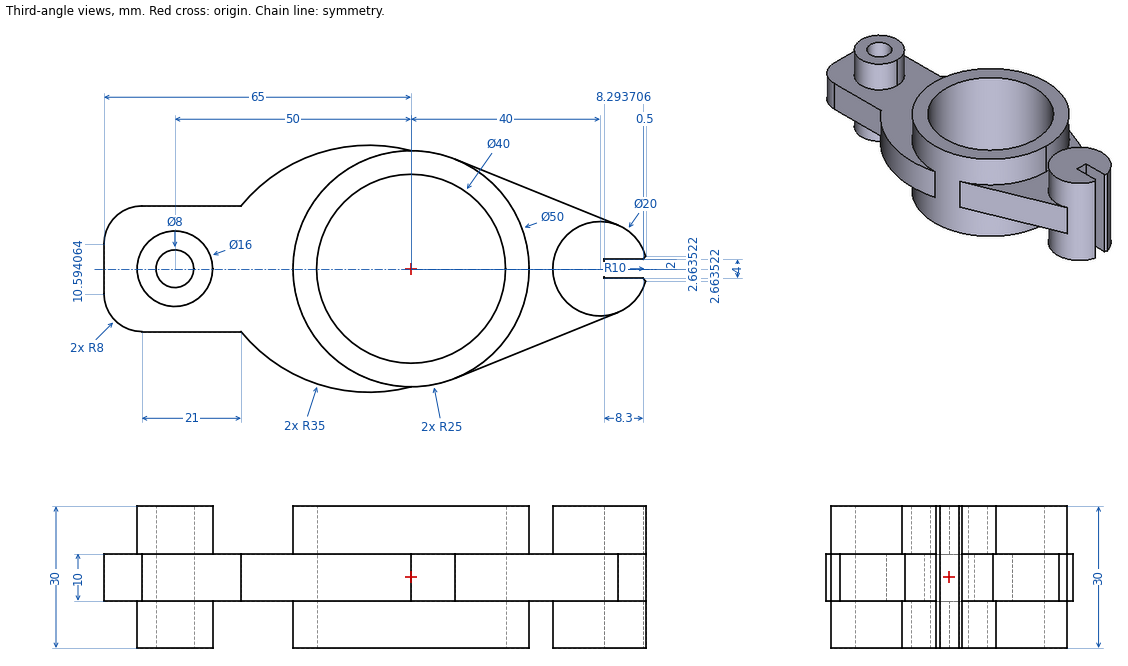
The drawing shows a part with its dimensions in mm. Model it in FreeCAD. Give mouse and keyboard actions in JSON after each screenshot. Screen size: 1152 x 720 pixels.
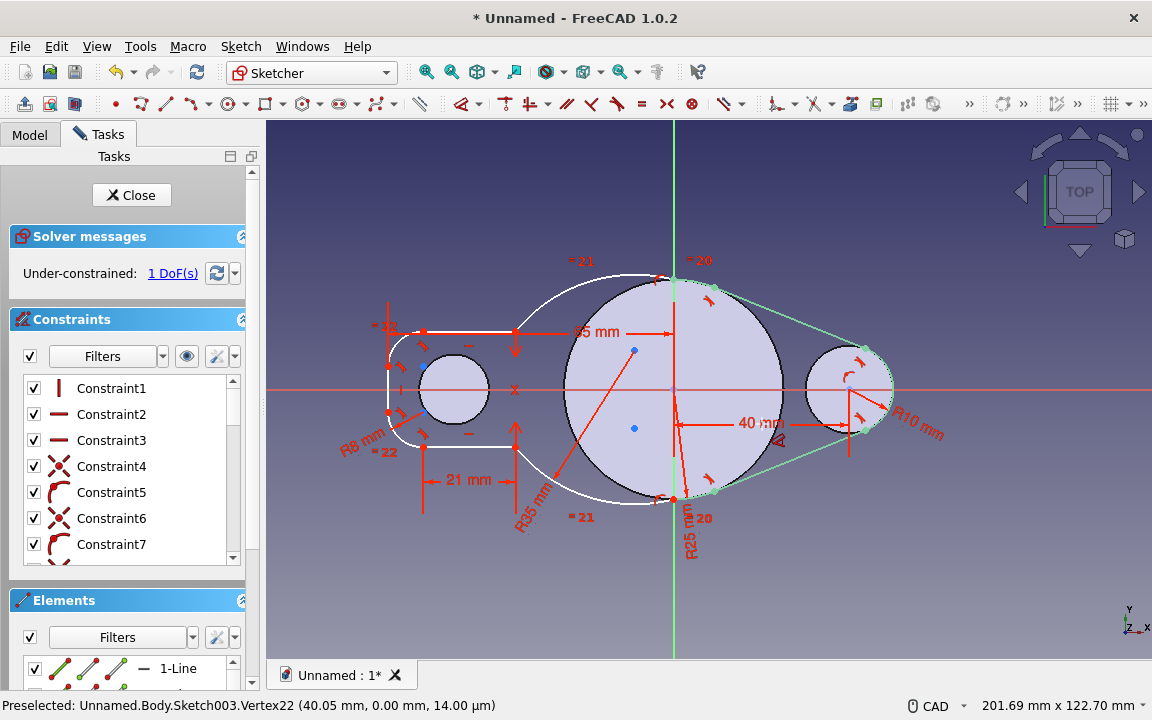
{"action": "scroll", "coordinate": [388, 380], "scroll_direction": "up", "scroll_amount": 3}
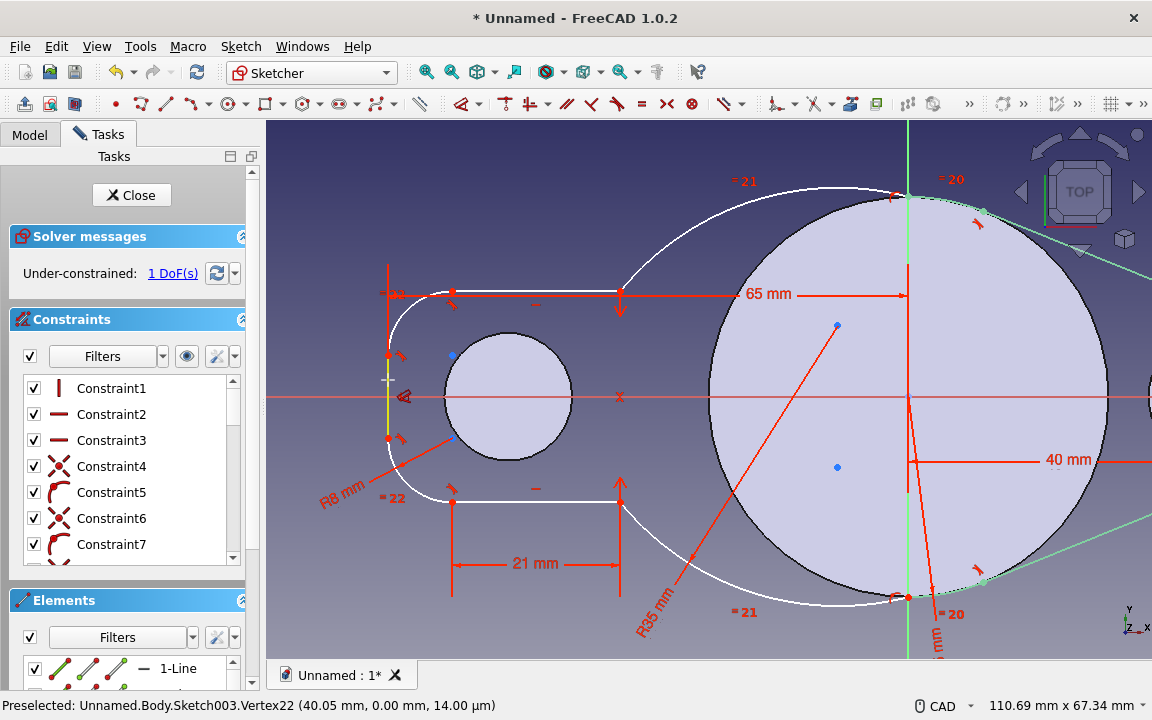
{"action": "left_click", "coordinate": [388, 380]}
{"action": "left_click", "coordinate": [354, 378]}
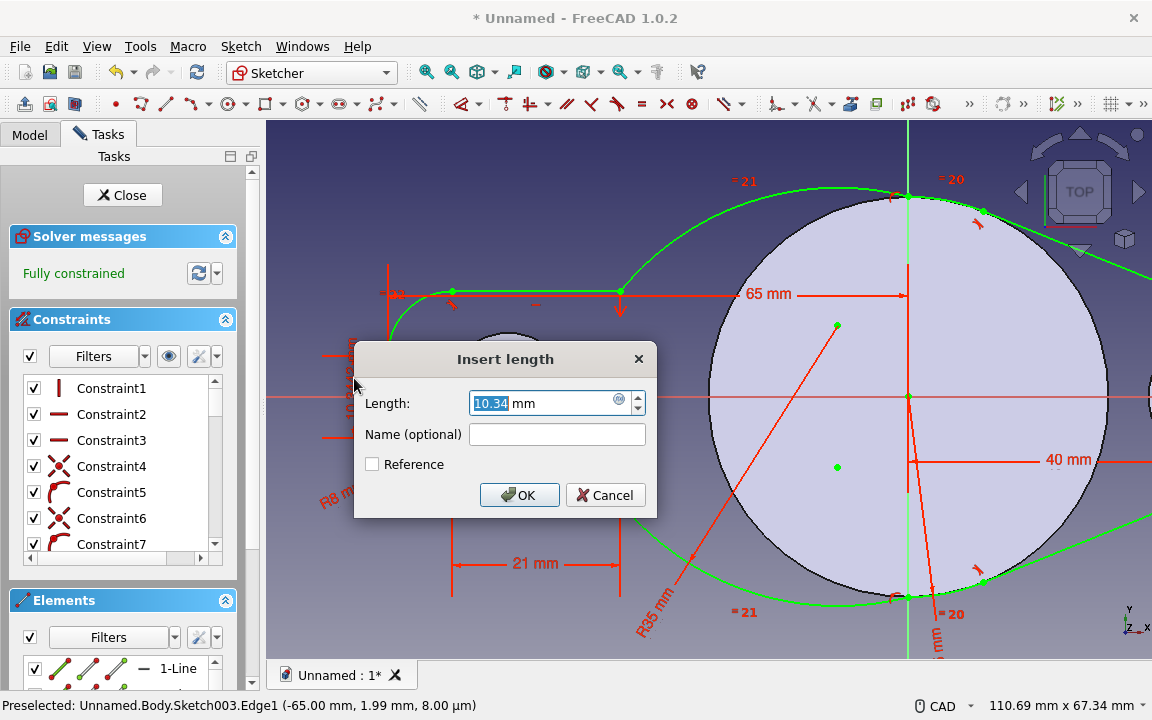
{"action": "type", "text": "10.594064"}
{"action": "key", "text": "Return"}
{"action": "key", "text": "Escape"}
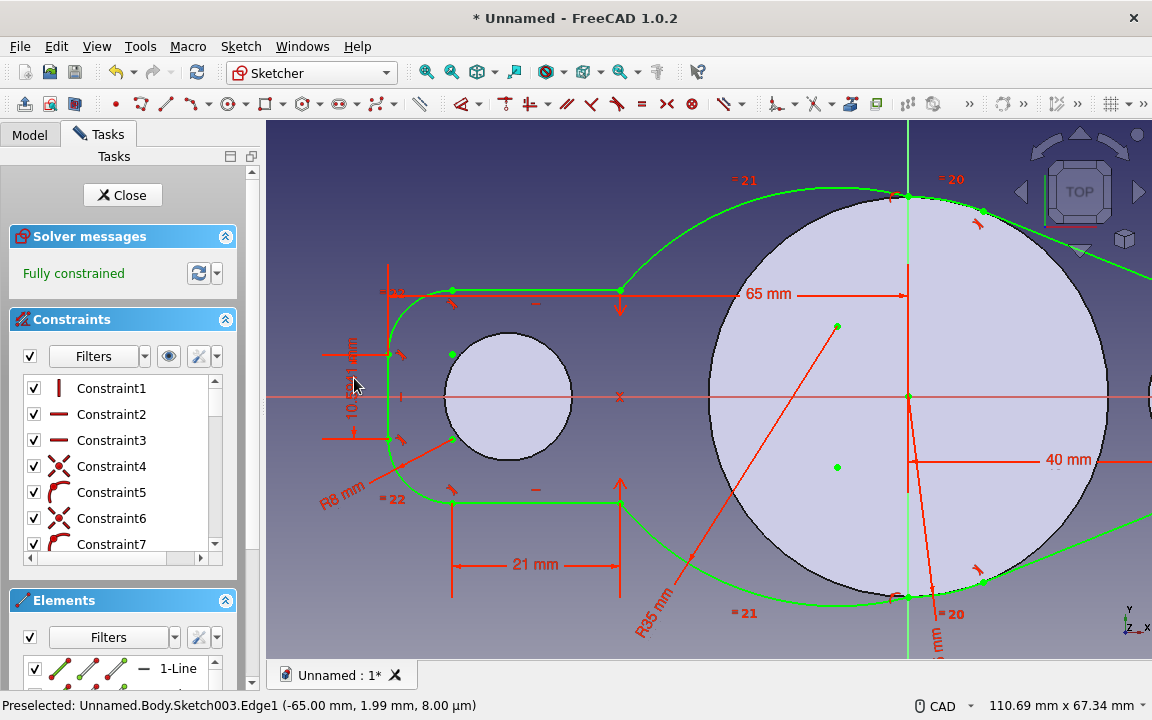
{"action": "left_click", "coordinate": [123, 195]}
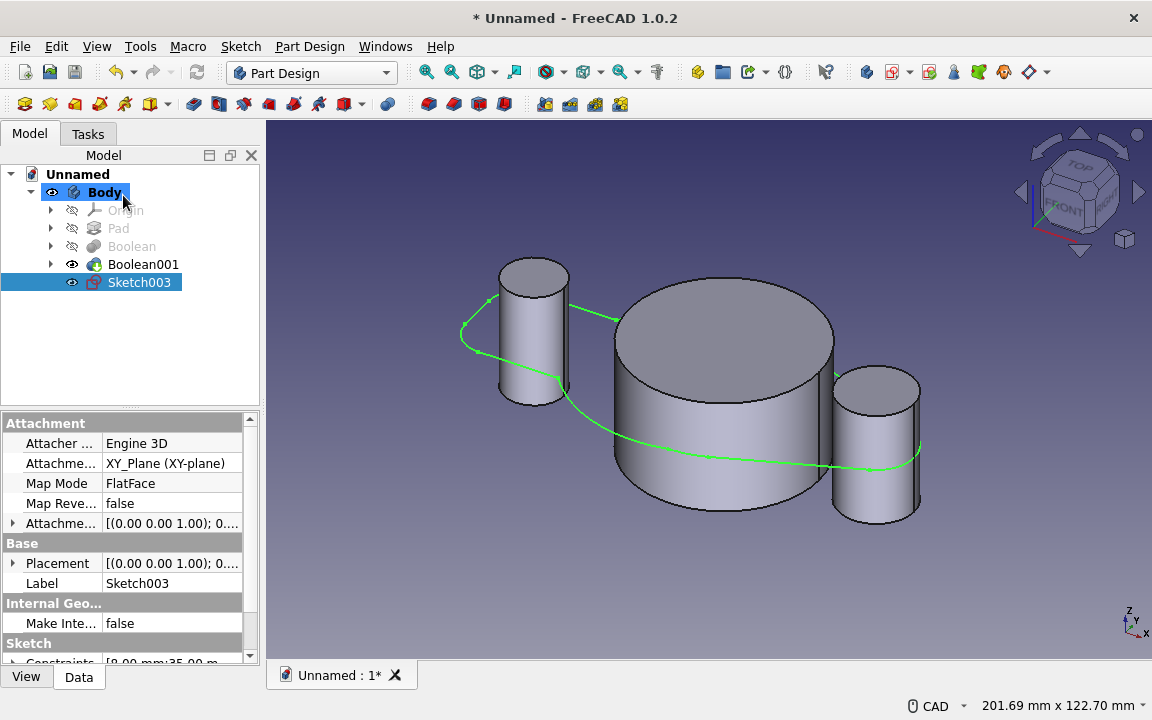
{"action": "left_click", "coordinate": [25, 104]}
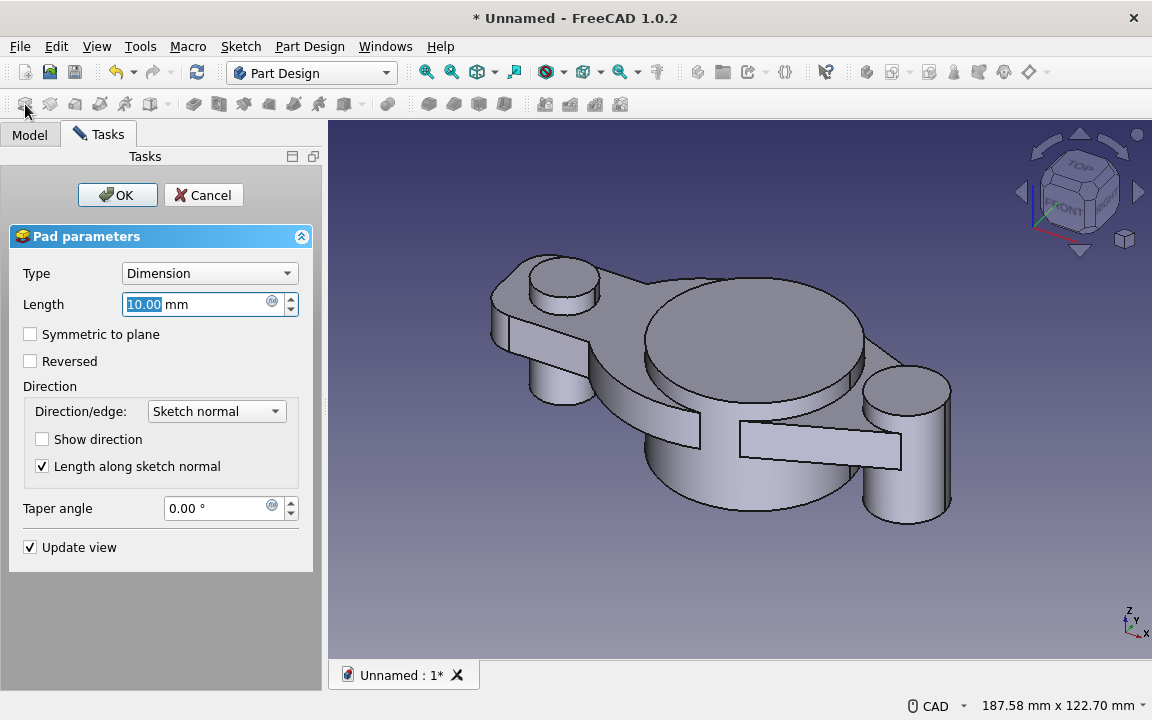
{"action": "type", "text": "10"}
{"action": "key", "text": "Tab"}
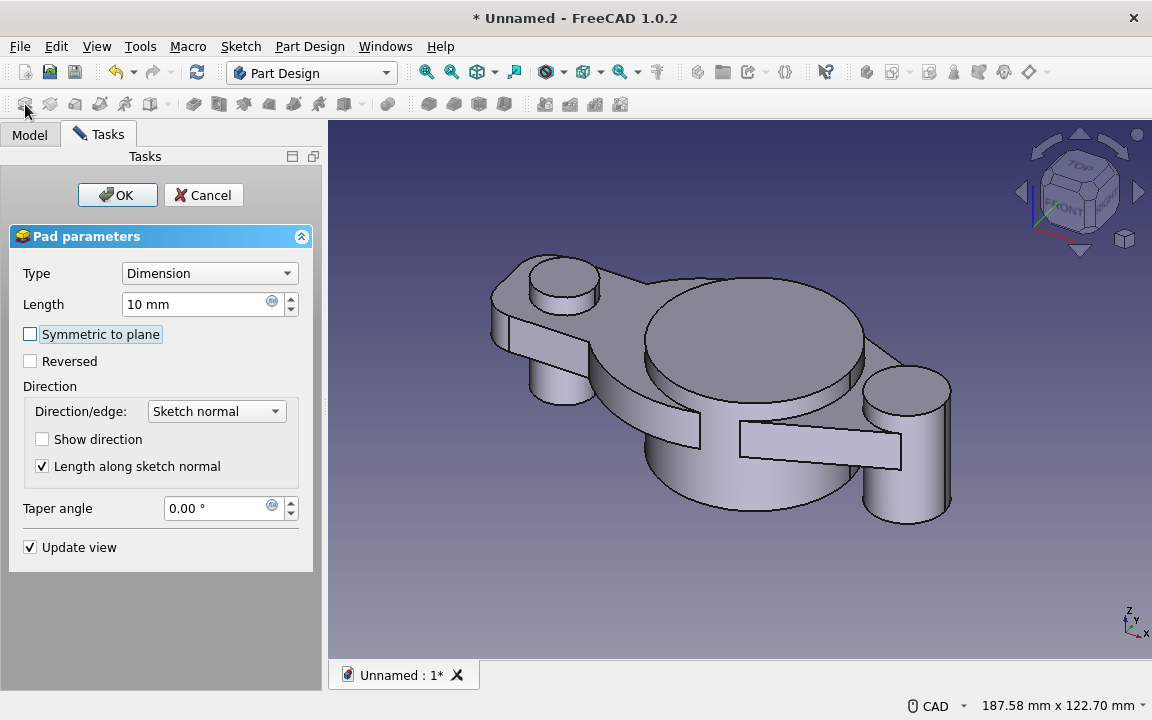
{"action": "left_click", "coordinate": [31, 334]}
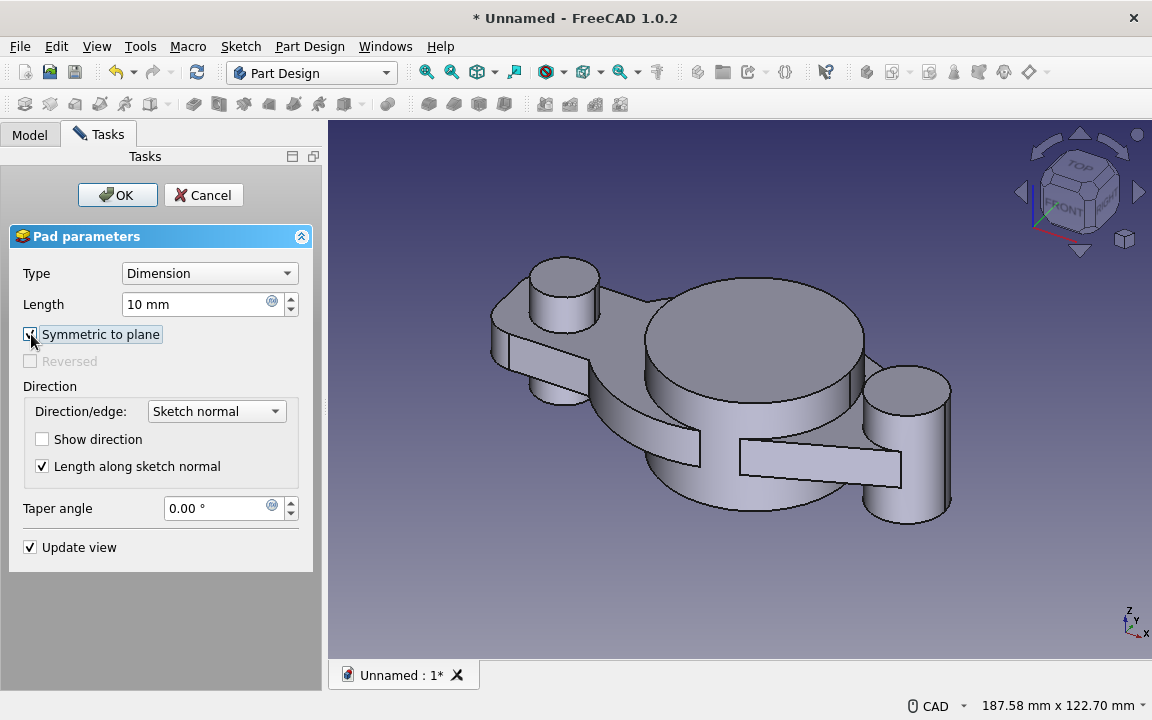
{"action": "left_click", "coordinate": [118, 195]}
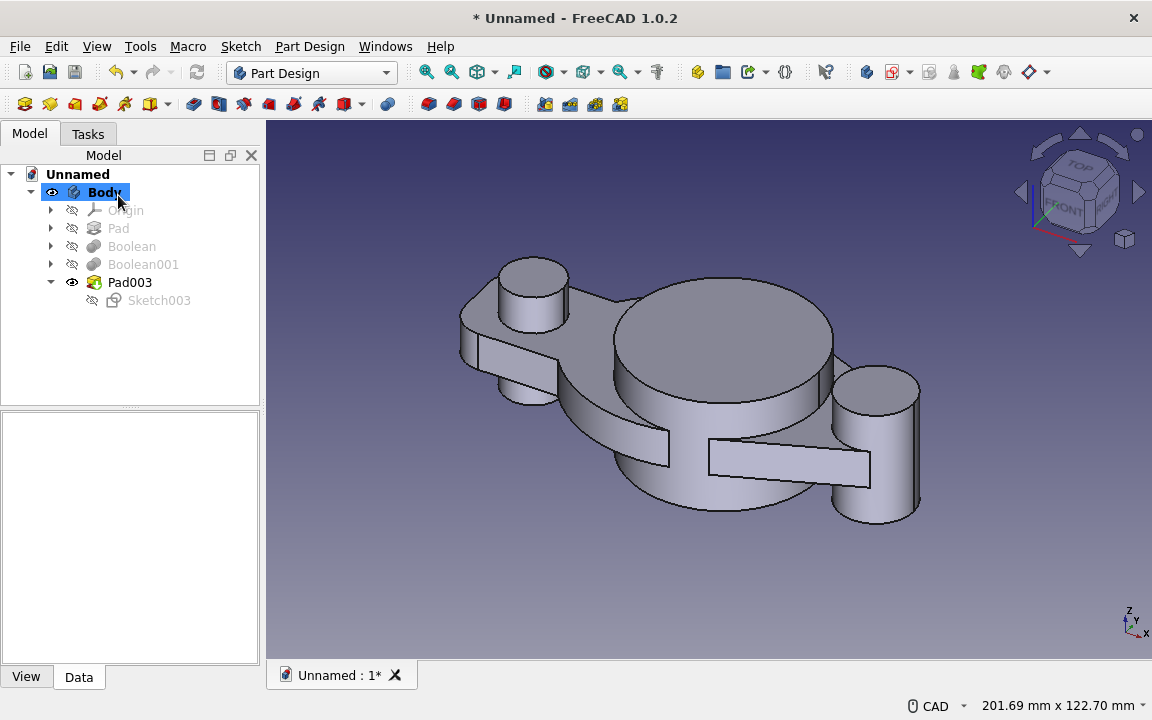
{"action": "left_click", "coordinate": [724, 339]}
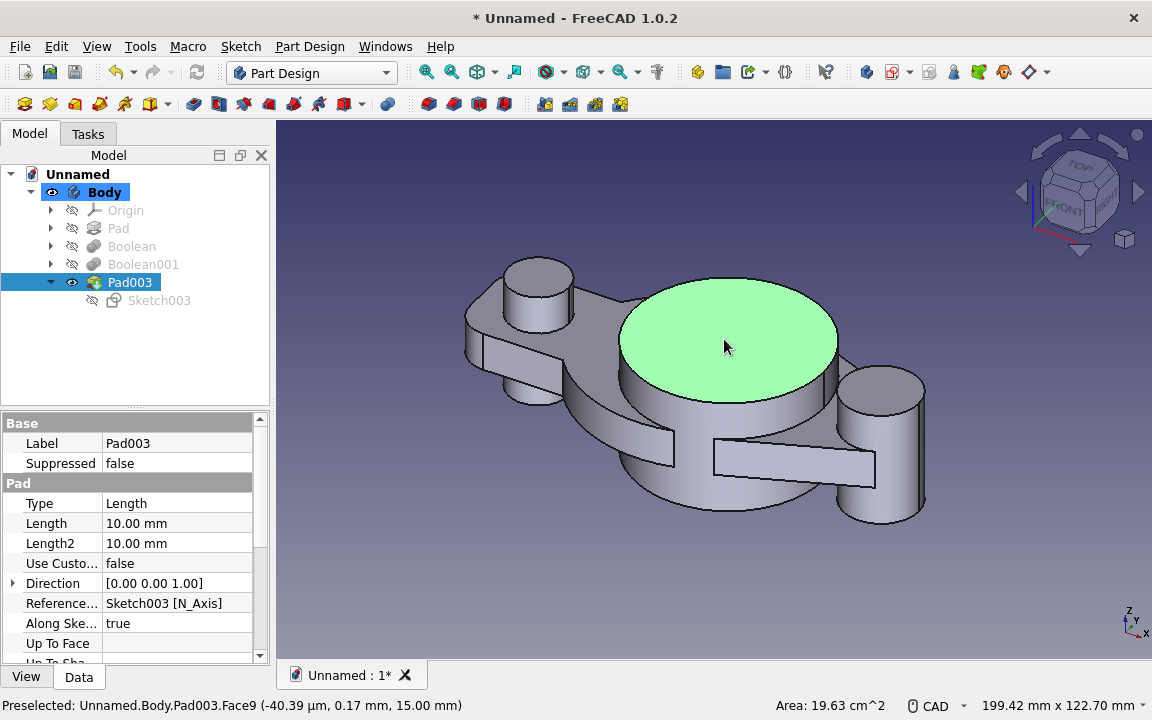
{"action": "left_click", "coordinate": [892, 72]}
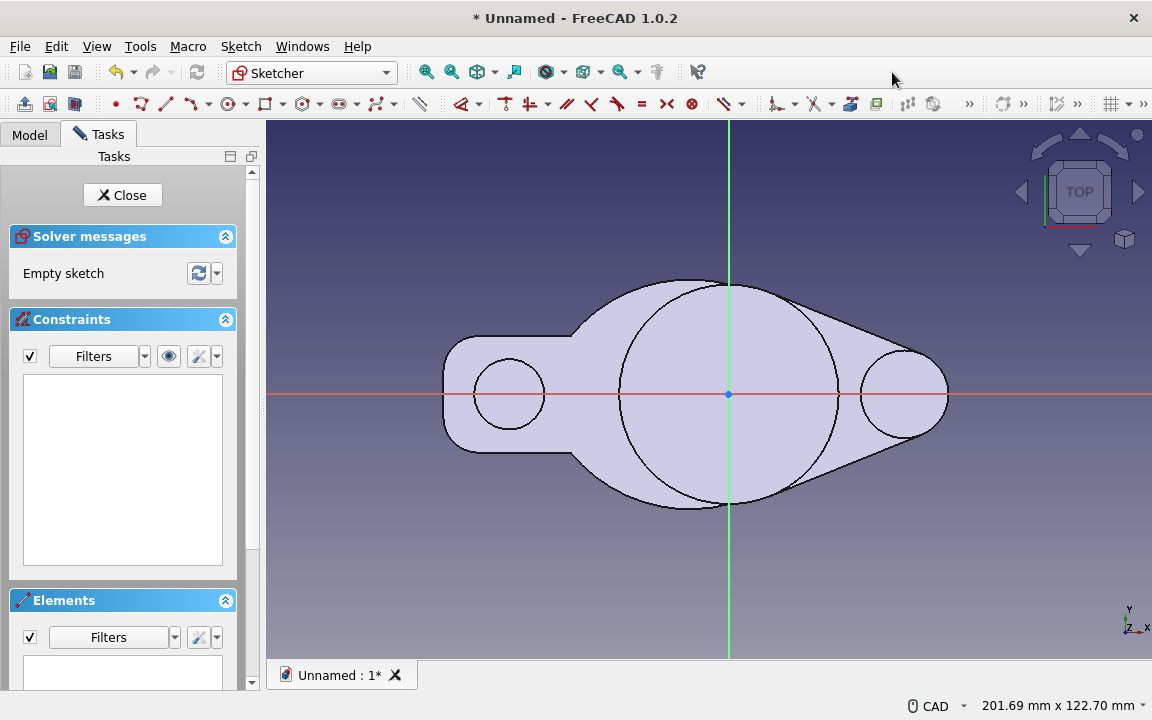
{"action": "left_click", "coordinate": [141, 104]}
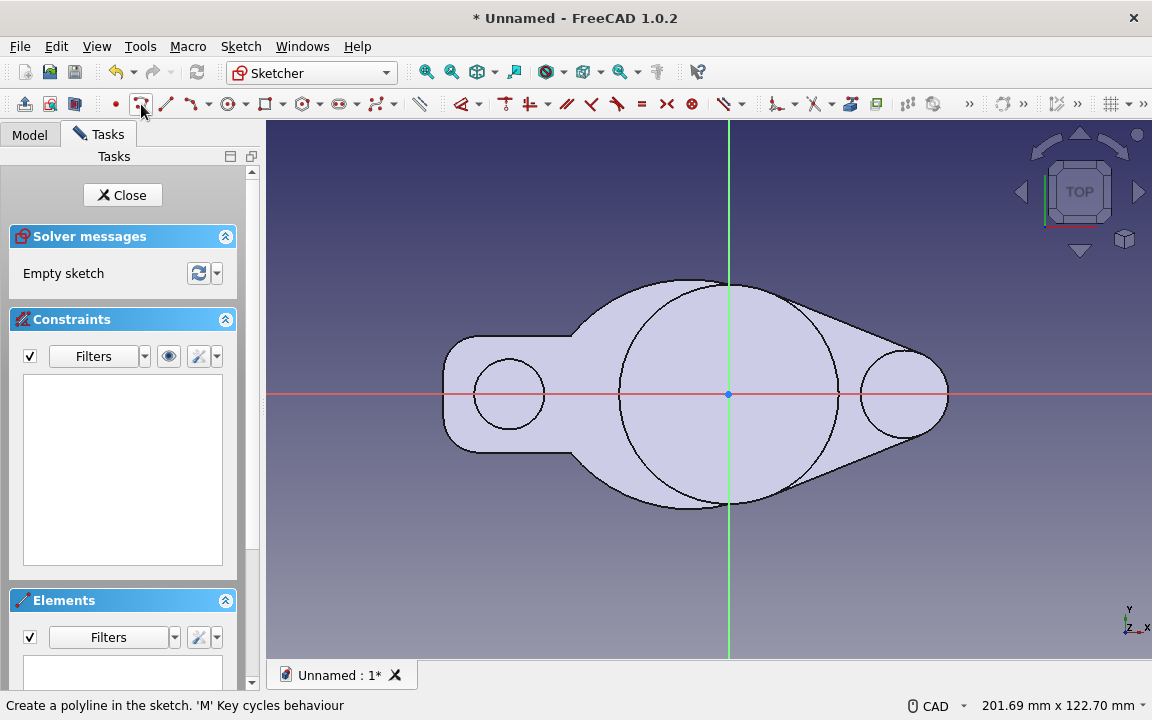
{"action": "scroll", "coordinate": [947, 383], "scroll_direction": "up", "scroll_amount": 2}